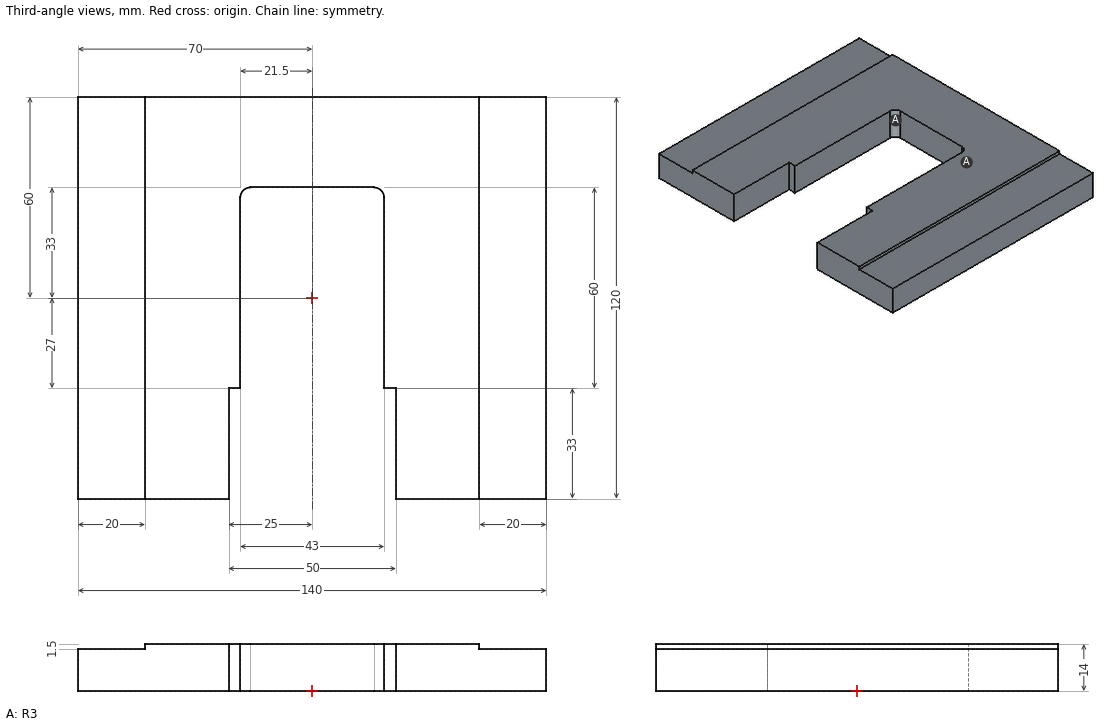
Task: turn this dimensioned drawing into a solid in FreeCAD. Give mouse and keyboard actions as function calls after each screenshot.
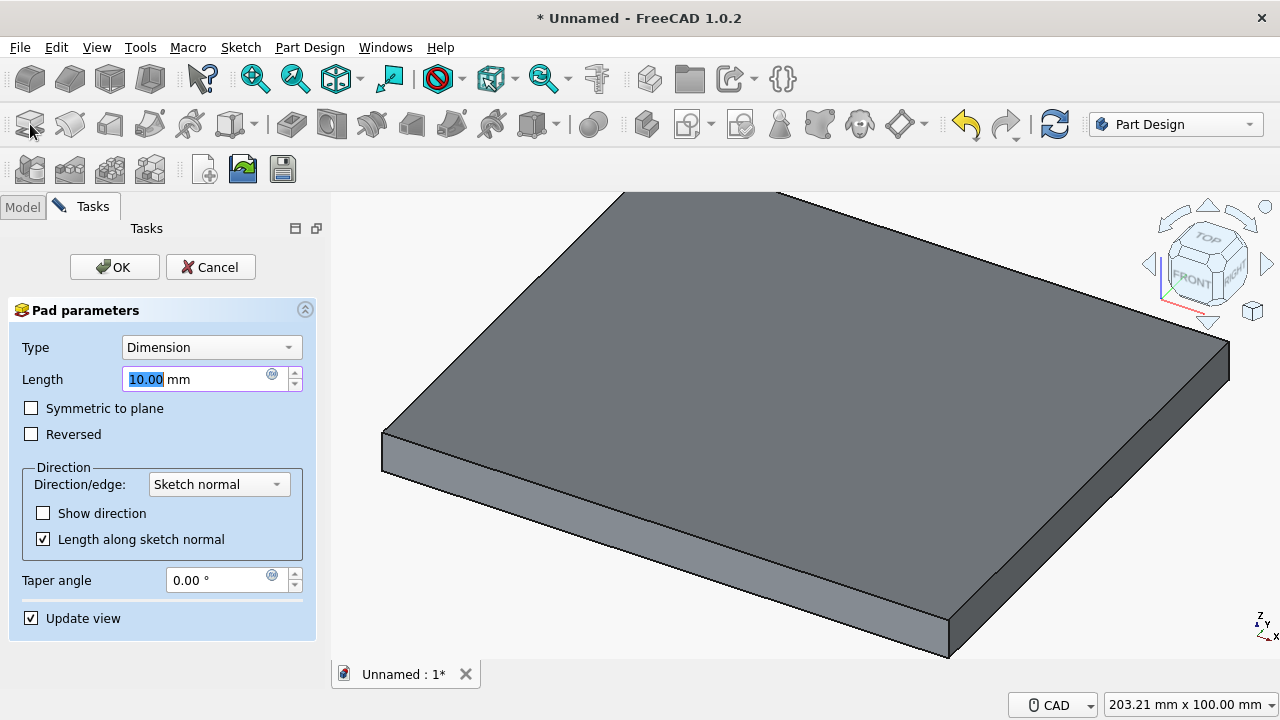
text(14)
key(Tab)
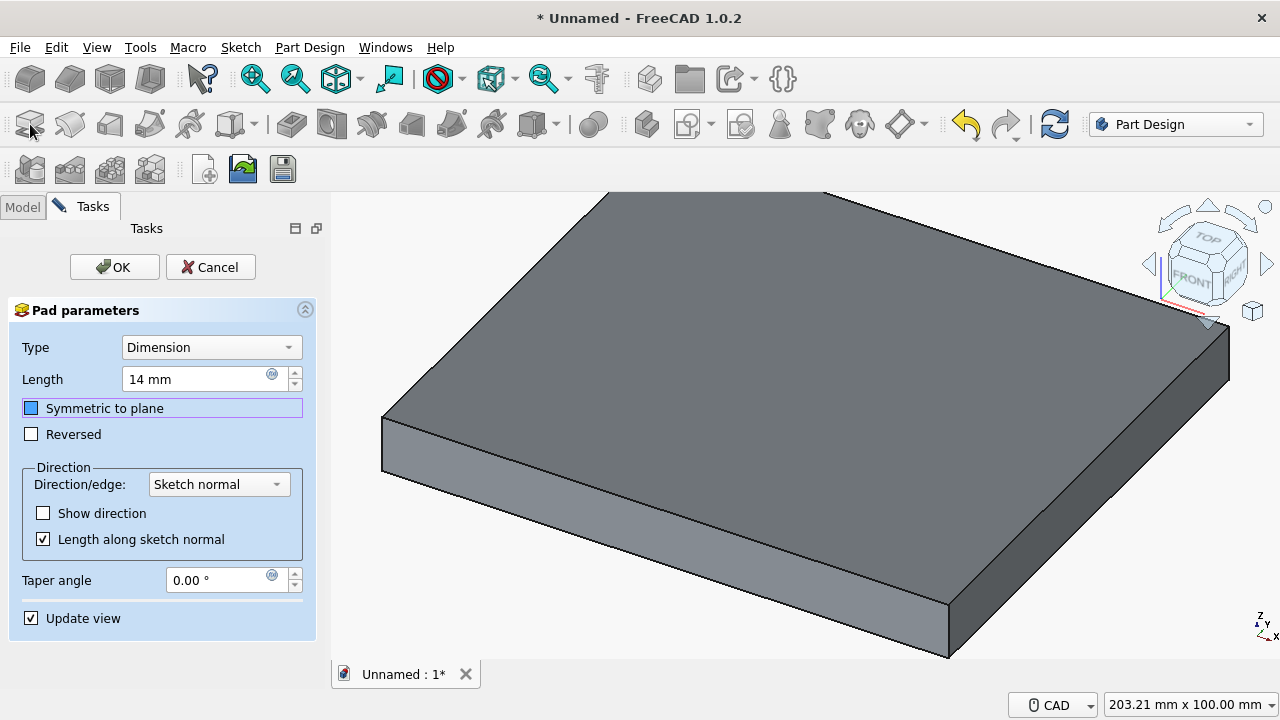
click(115, 267)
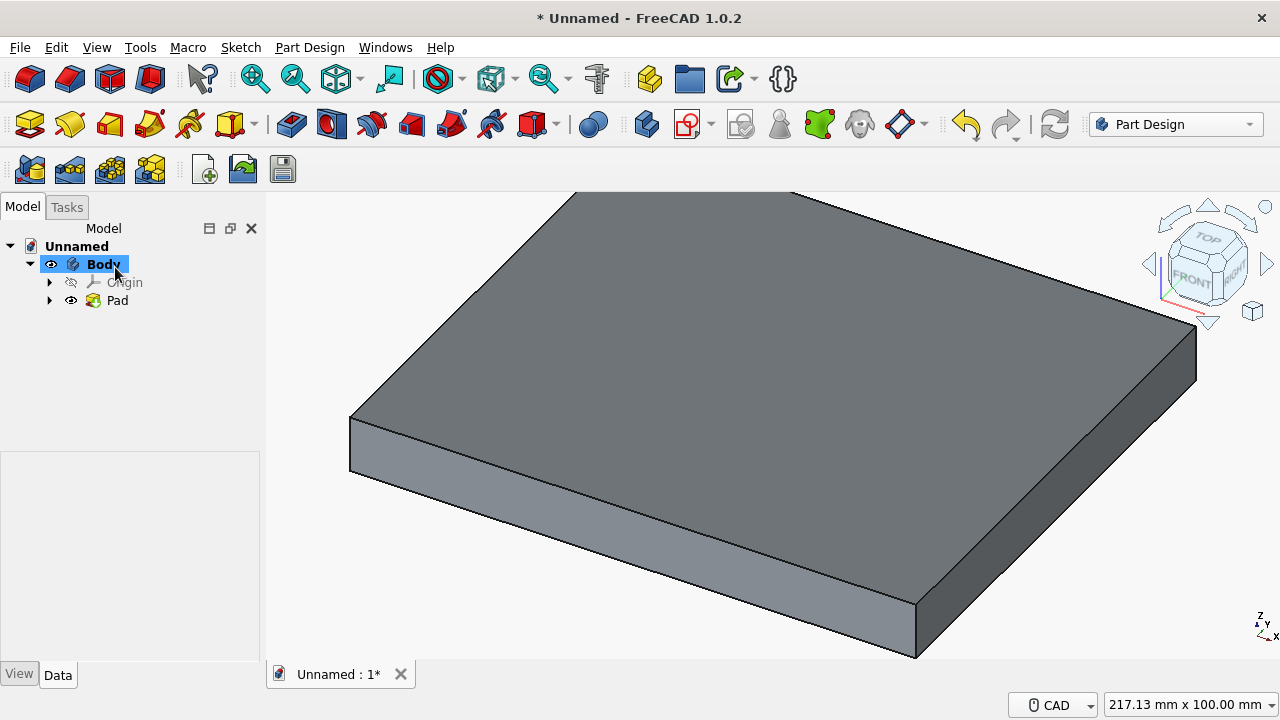
click(256, 80)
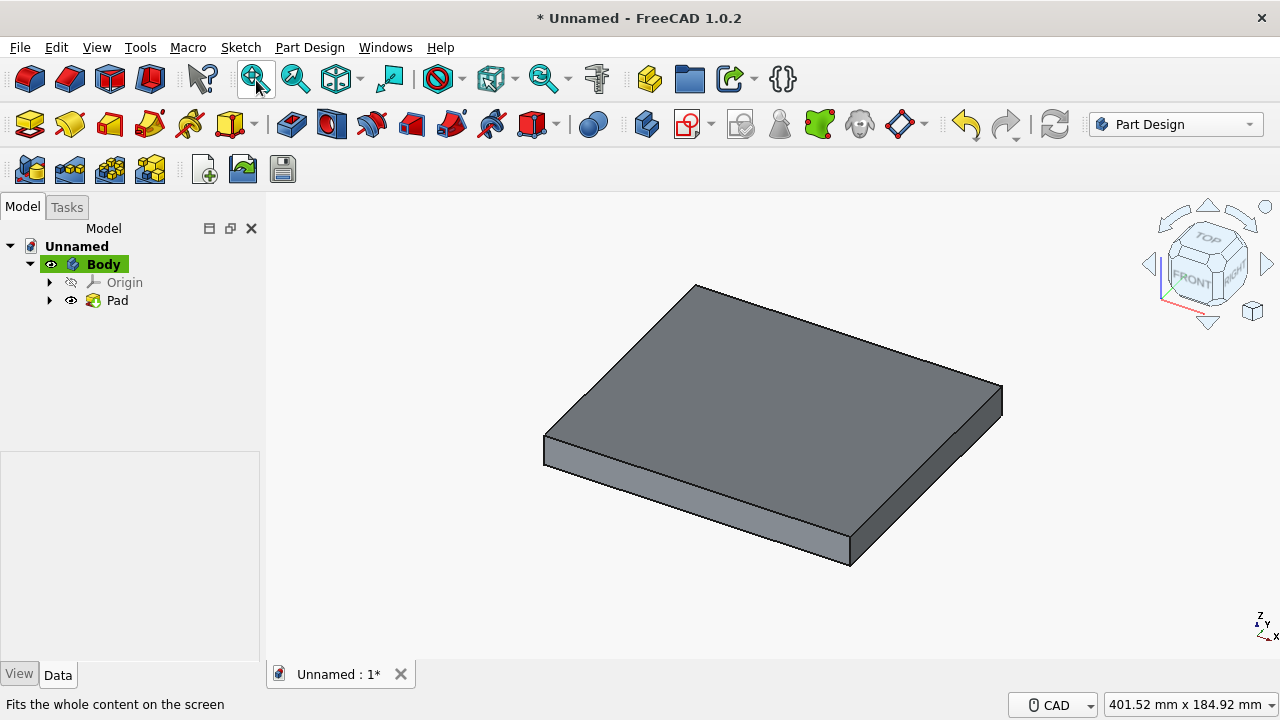
click(773, 410)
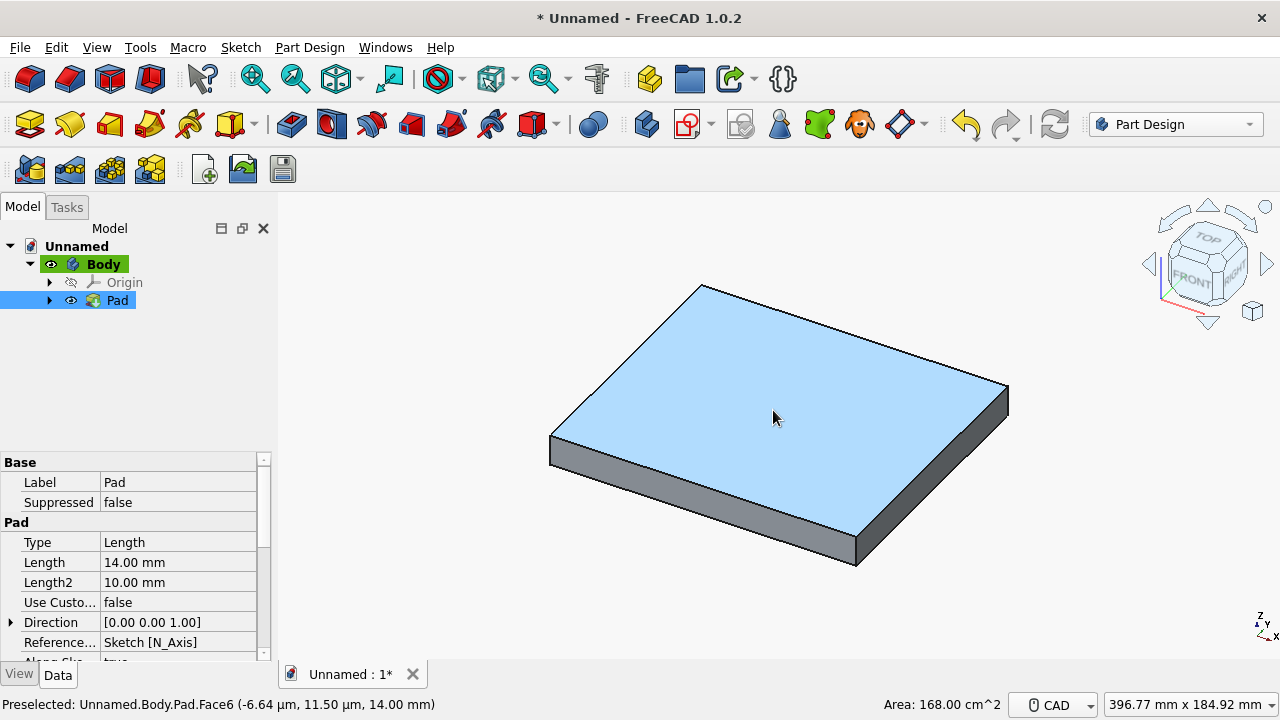
click(688, 124)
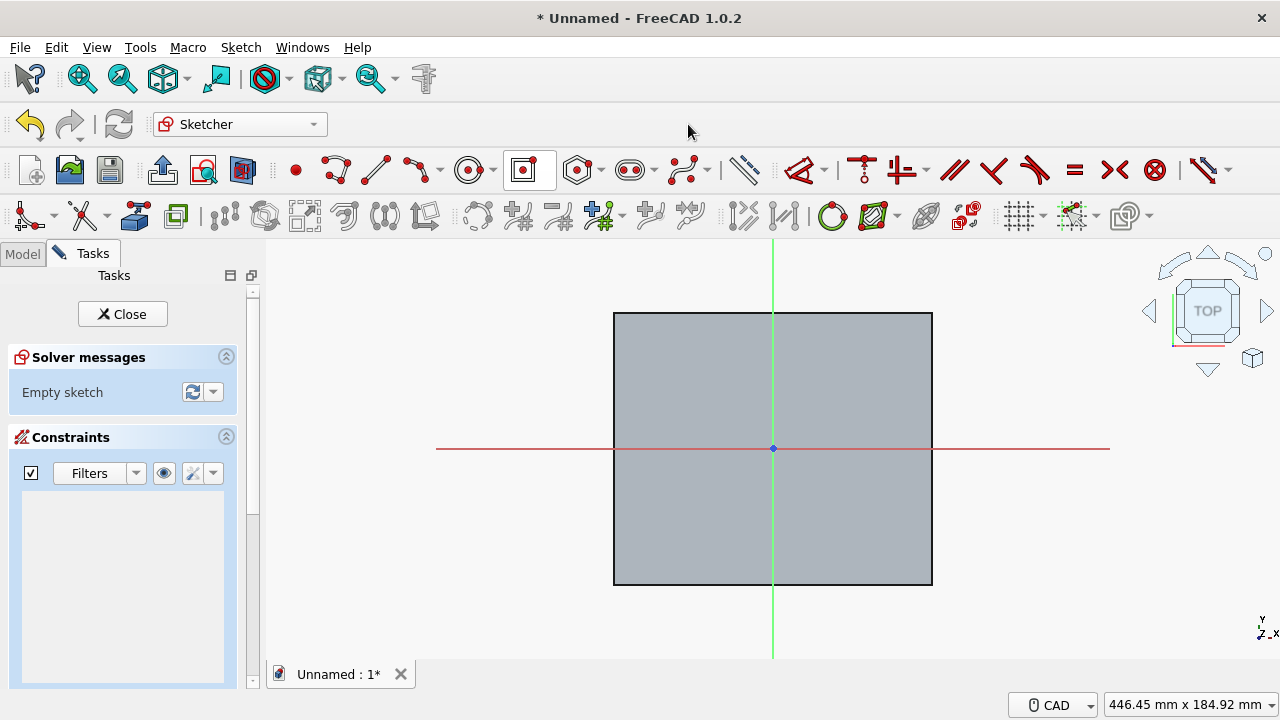
key(g)
key(r)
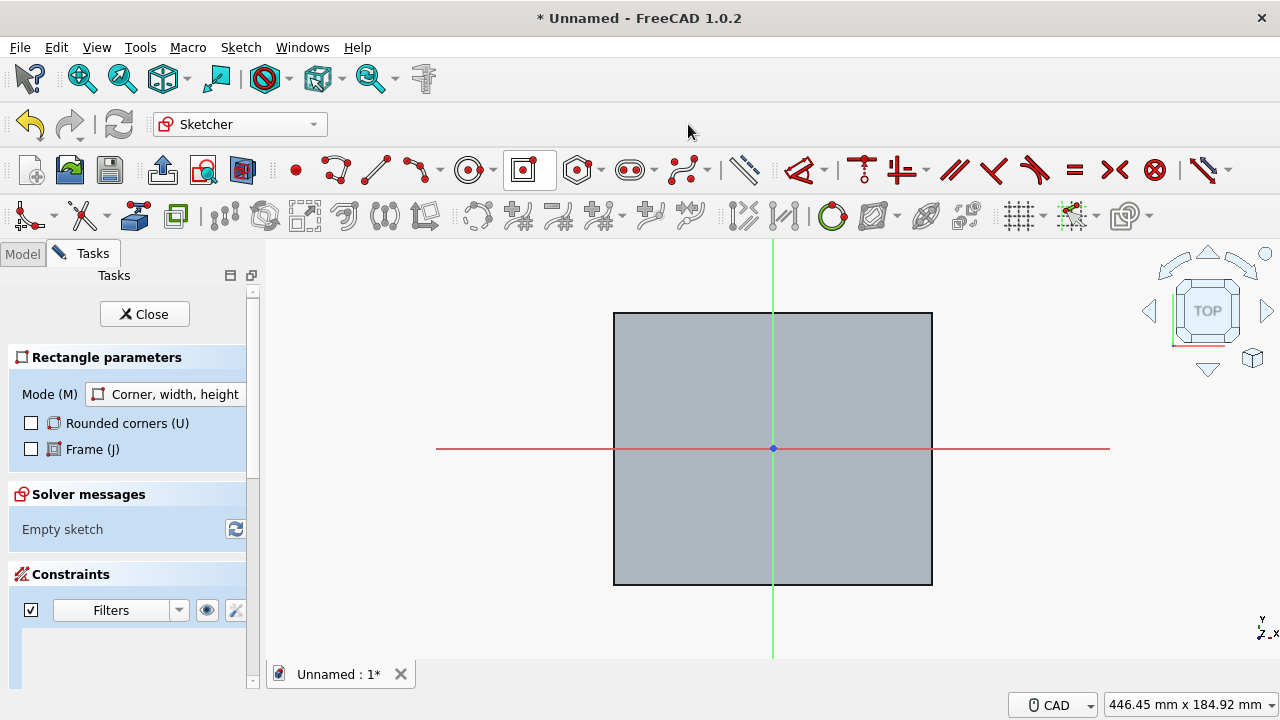
click(614, 313)
move(659, 585)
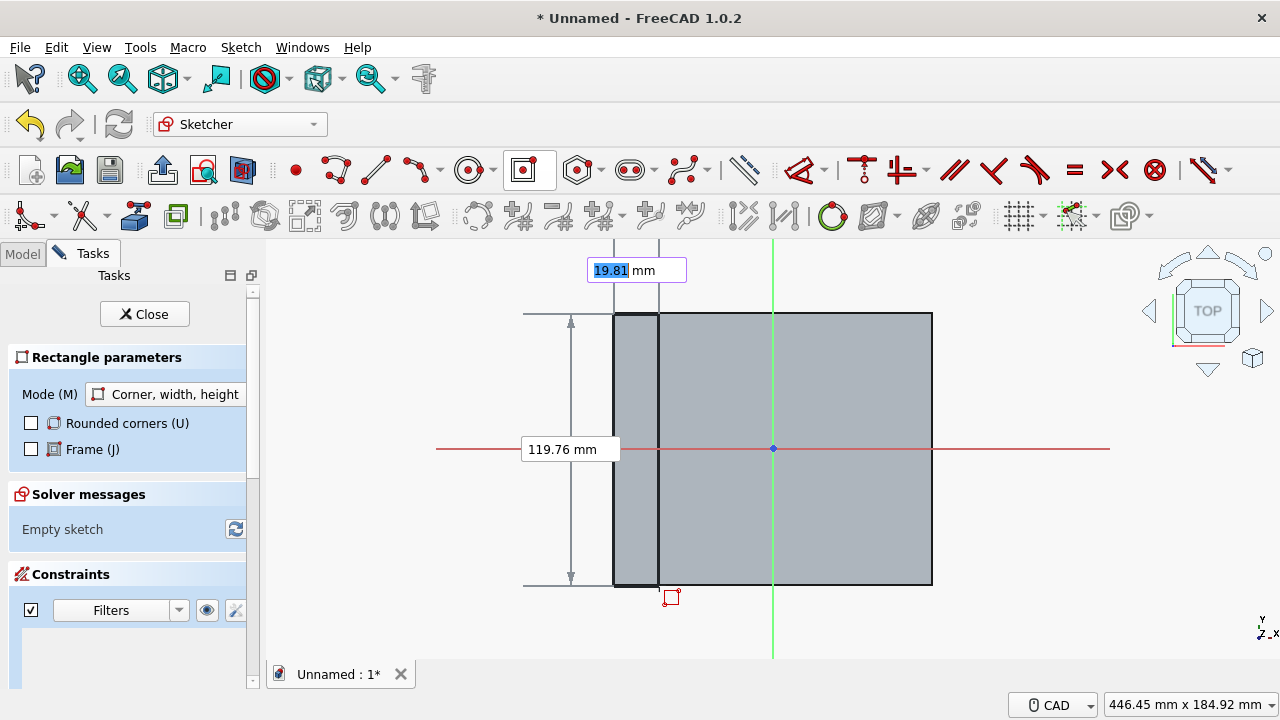
text(20)
key(Tab)
text(120)
key(Return)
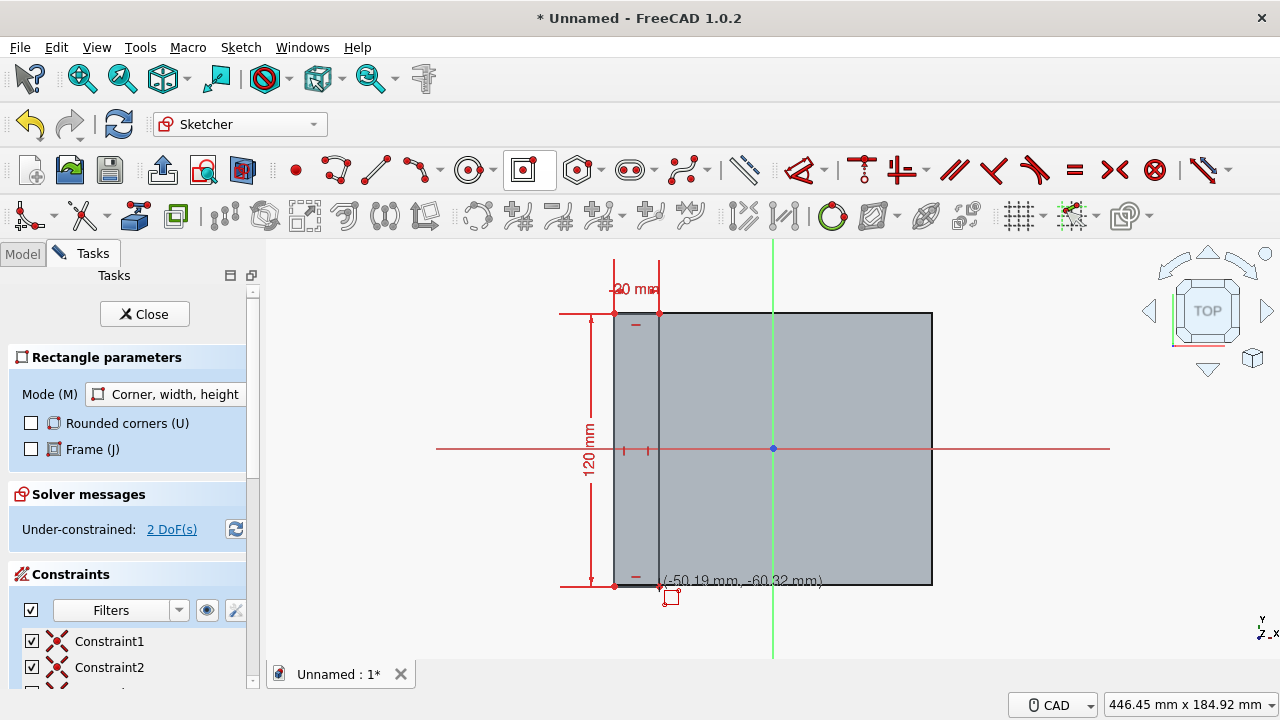
click(887, 313)
move(932, 585)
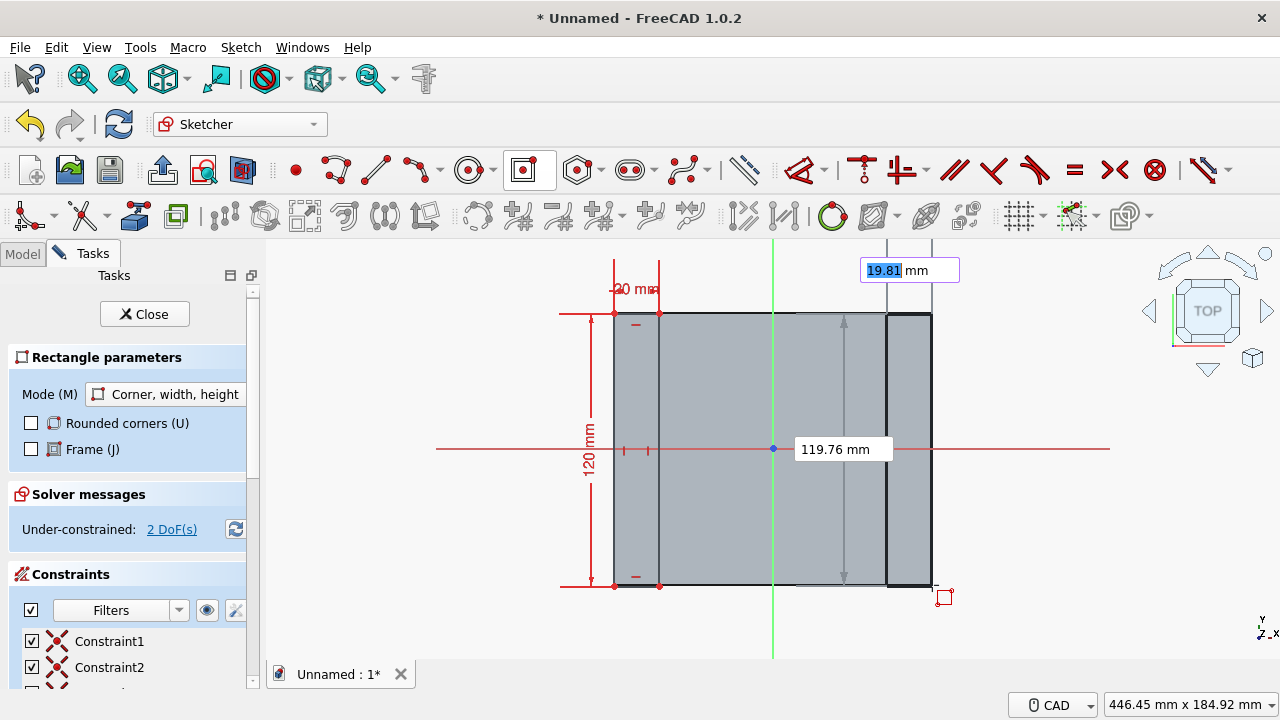
text(20)
key(Tab)
text(120)
key(Return)
key(Escape)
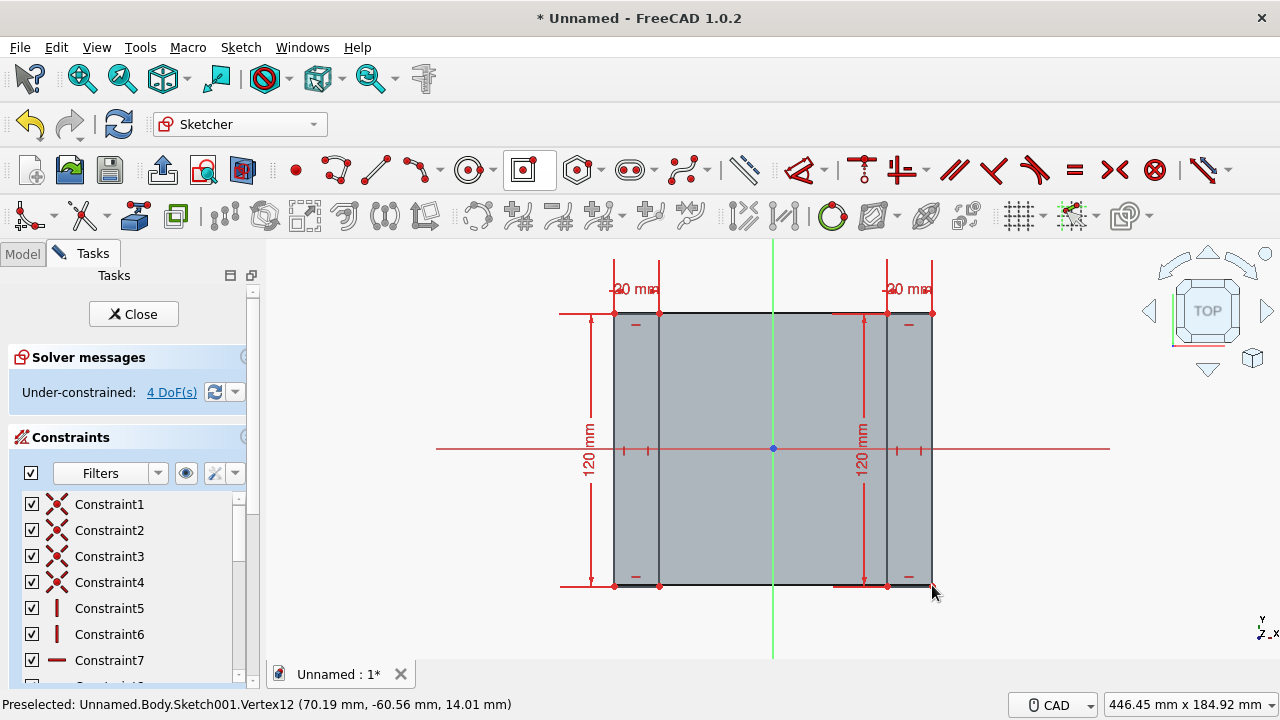
click(659, 314)